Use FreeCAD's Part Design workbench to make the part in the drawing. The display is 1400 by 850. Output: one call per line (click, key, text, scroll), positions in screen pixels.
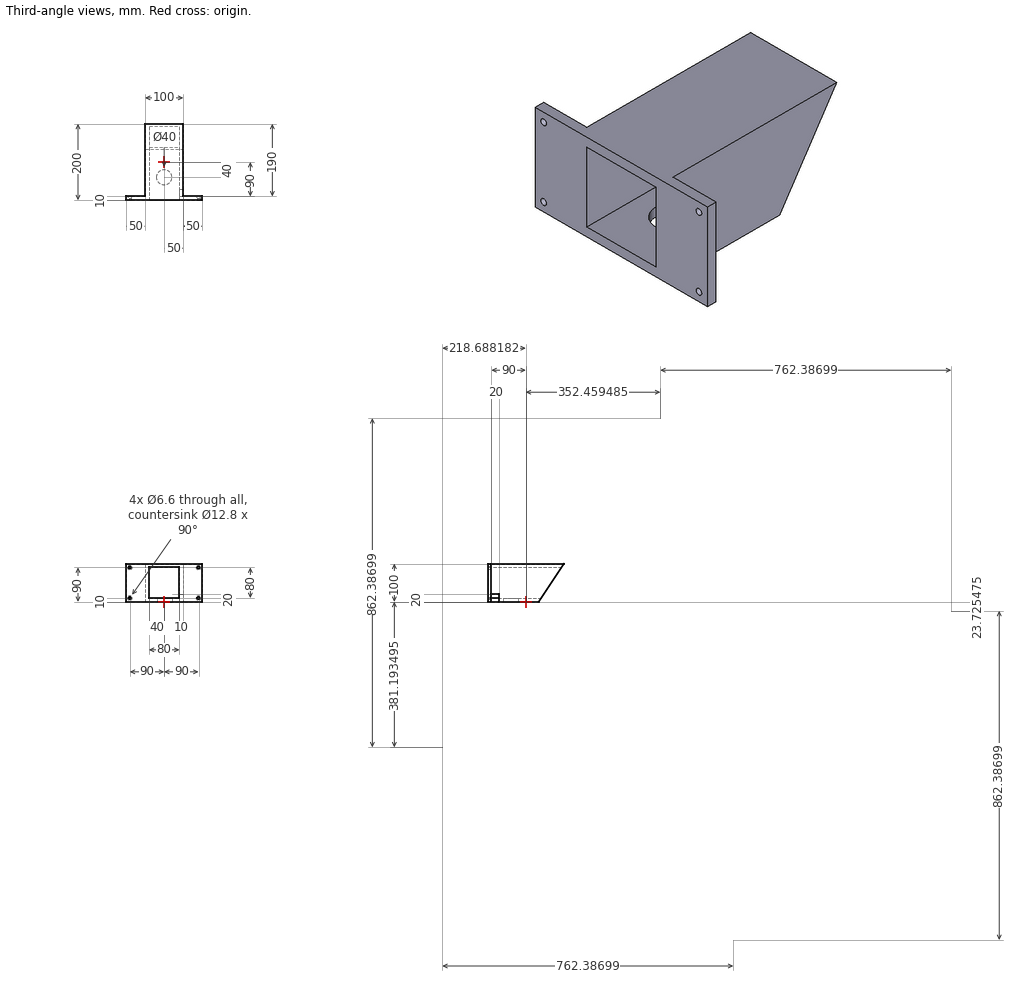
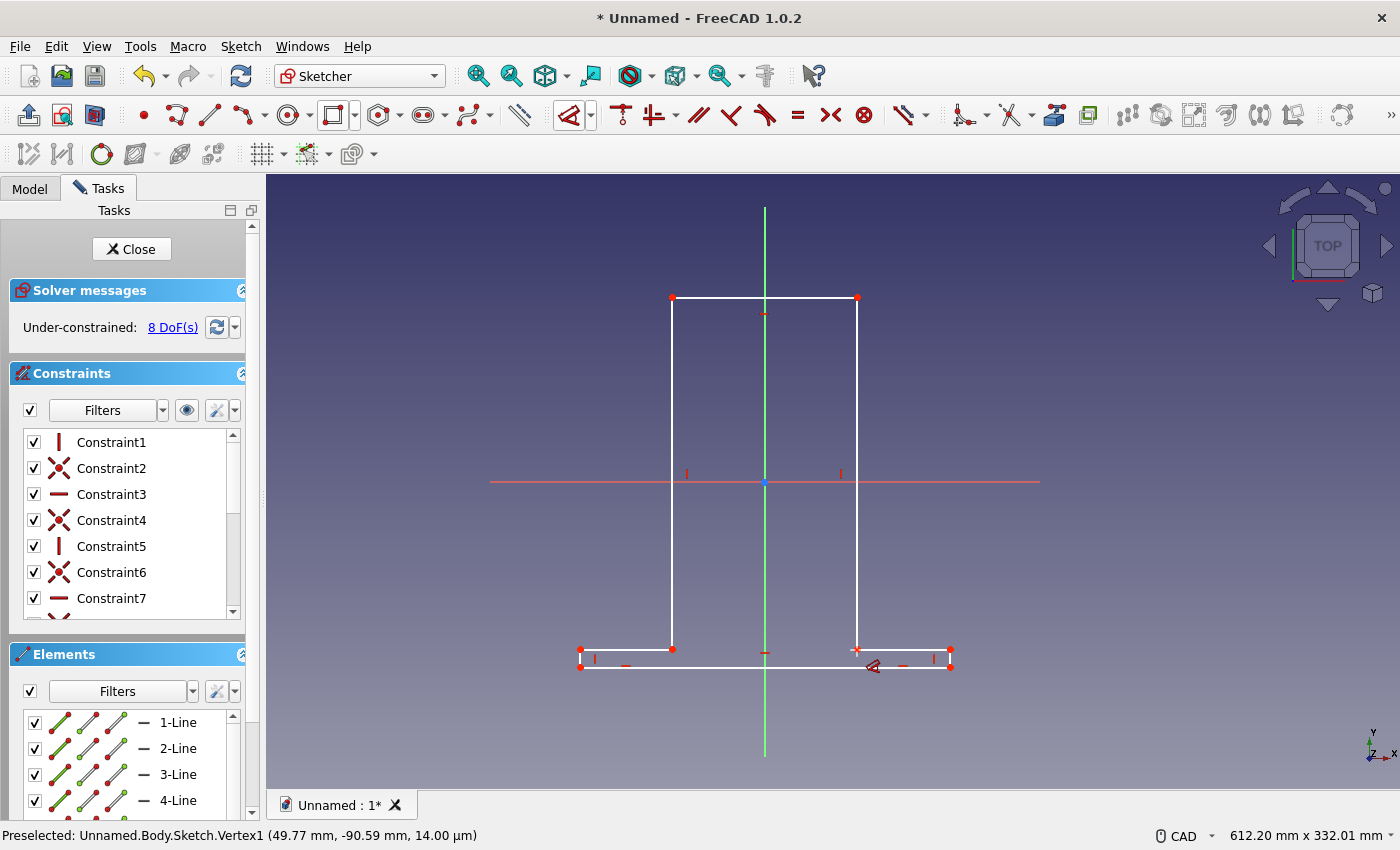
click(644, 650)
click(626, 684)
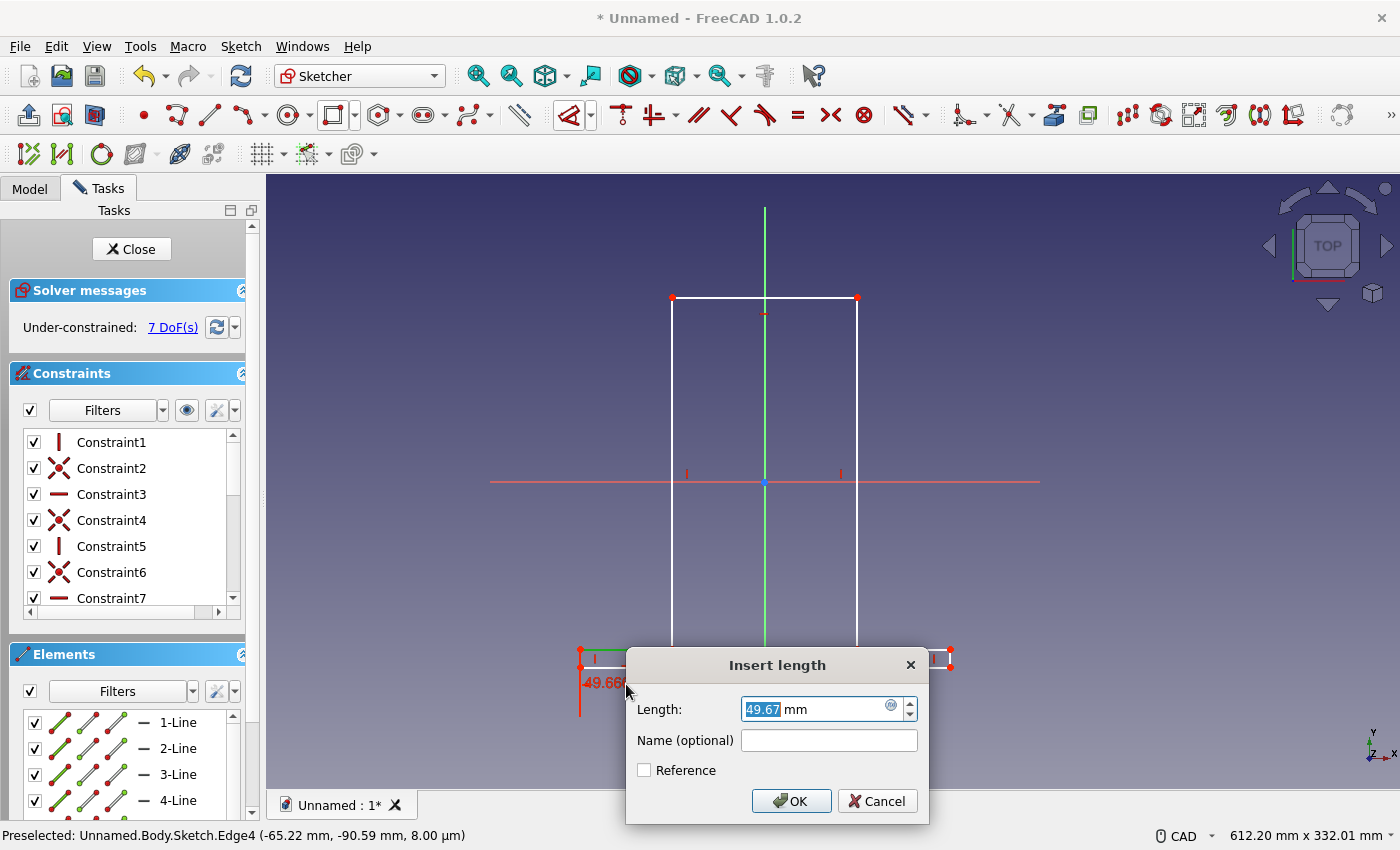
text(50)
key(Return)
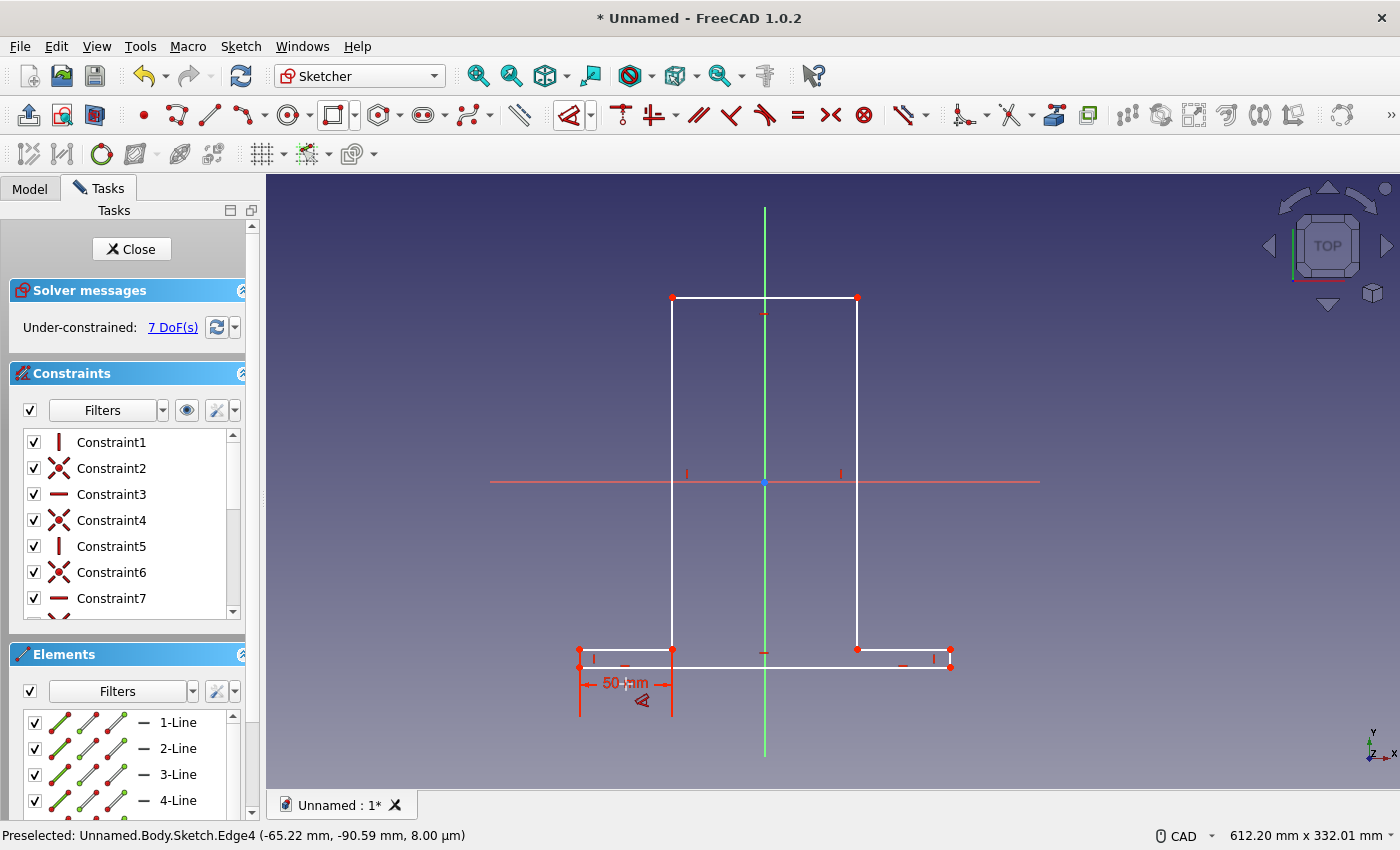
scroll(580, 659, up, 4)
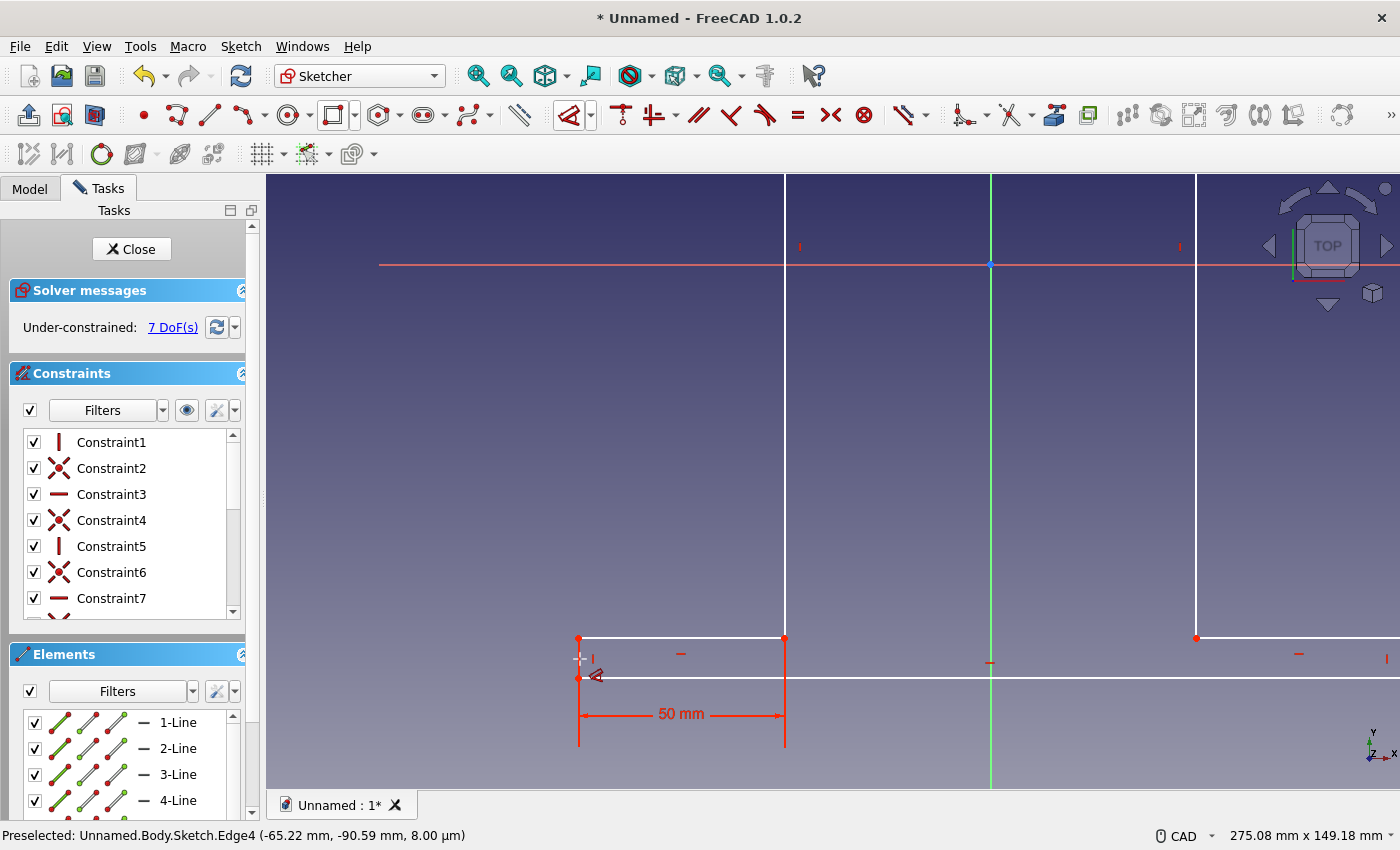
click(579, 658)
click(545, 658)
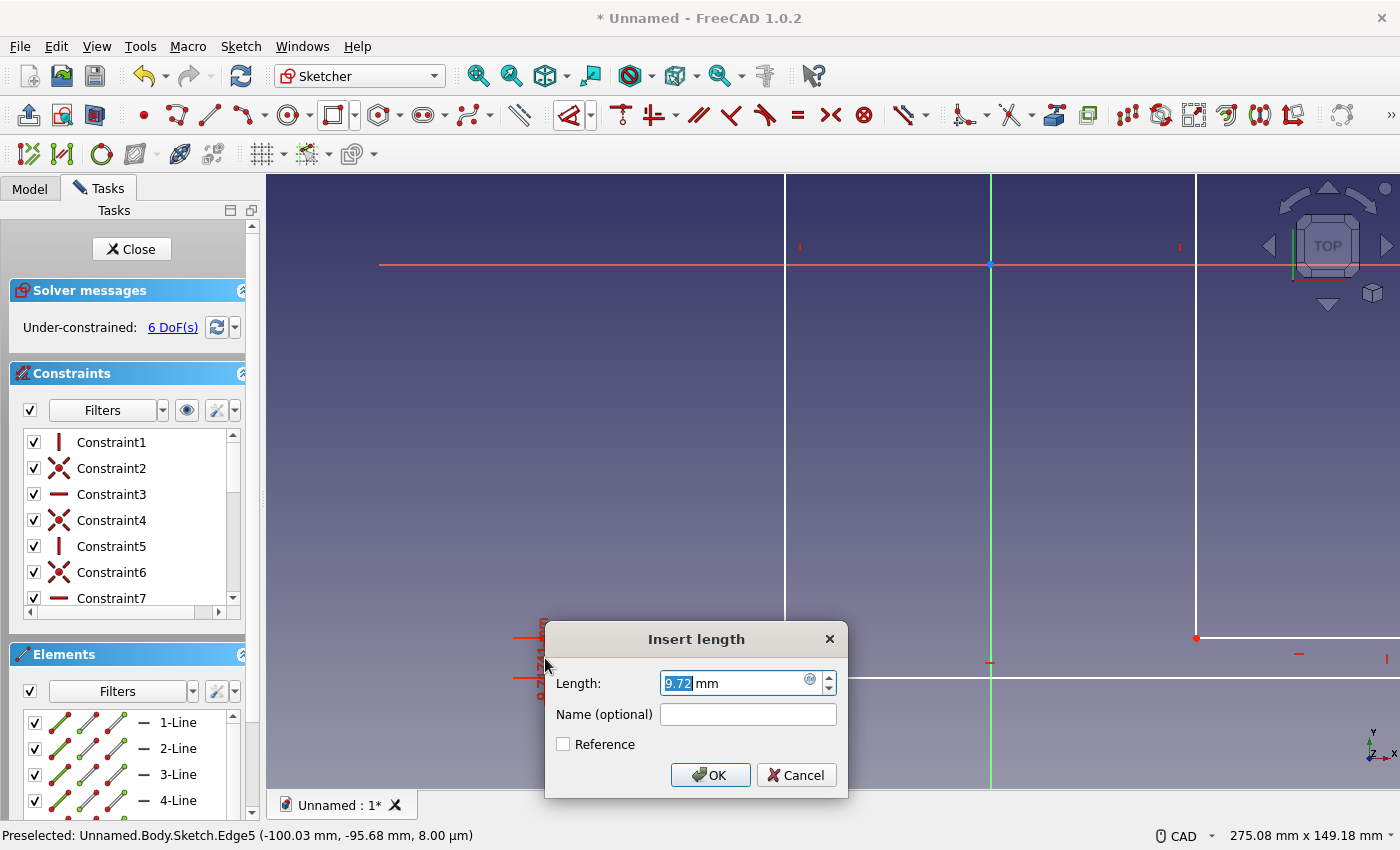
text(10)
key(Return)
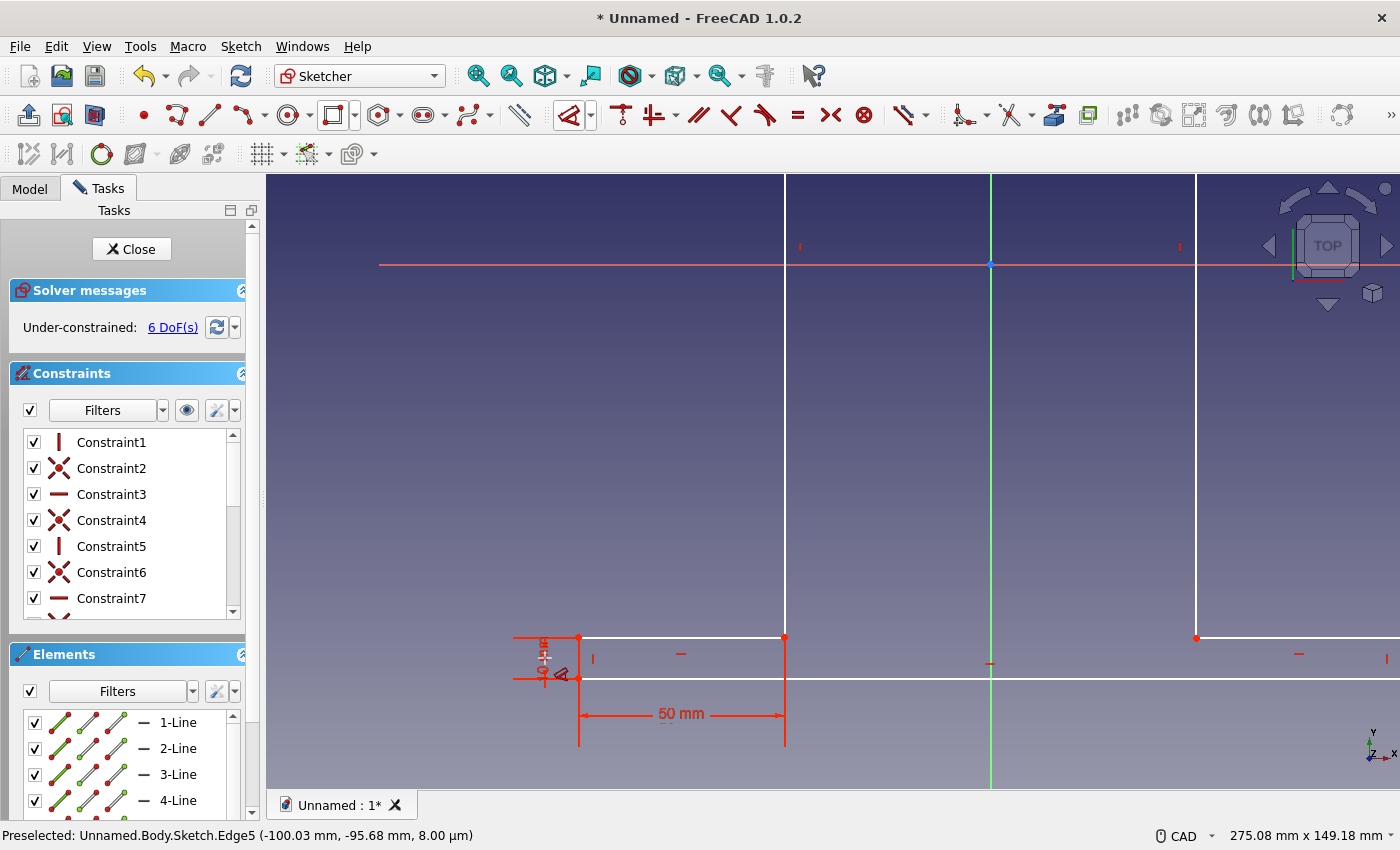
scroll(580, 659, down, 4)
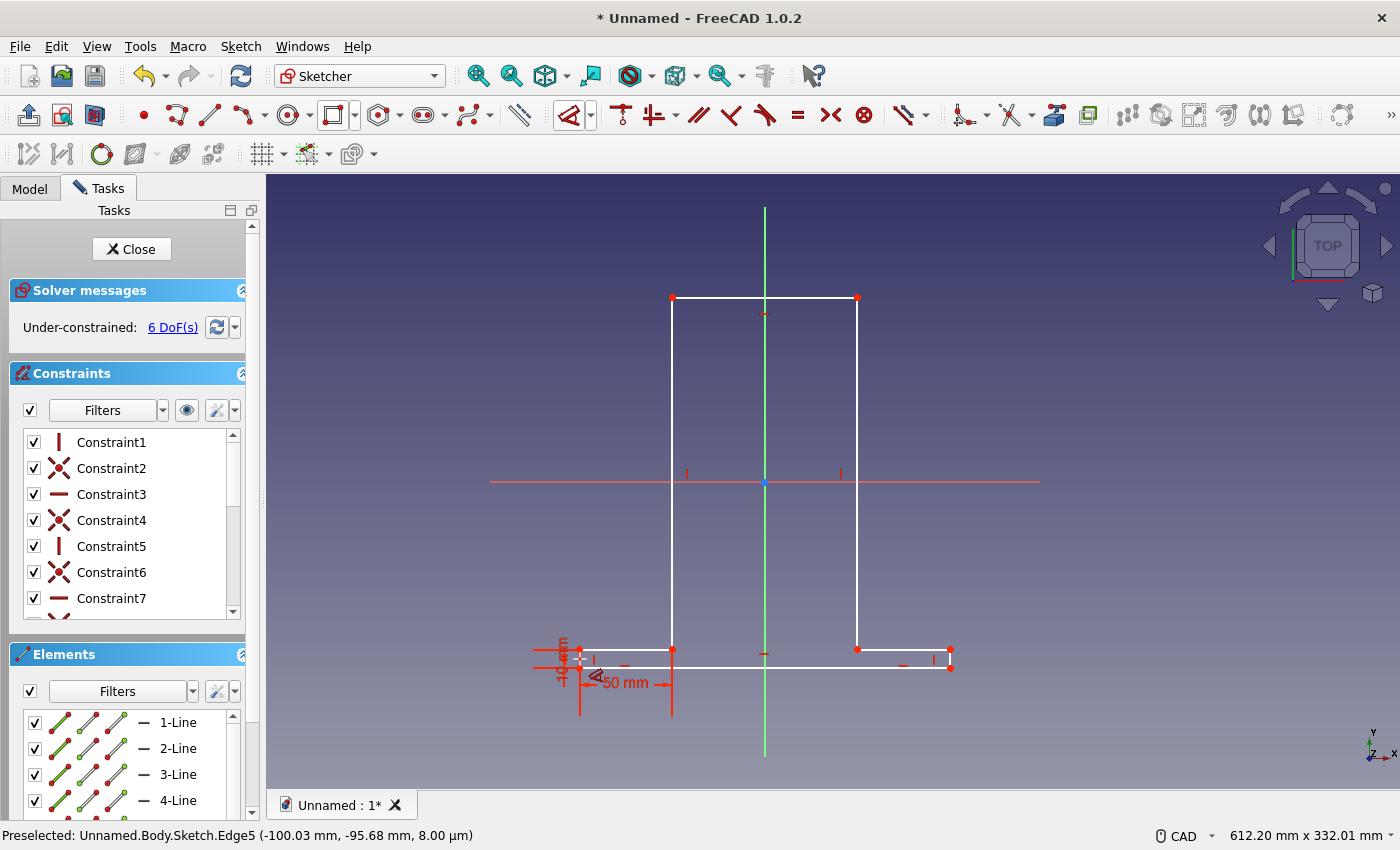
scroll(950, 663, up, 5)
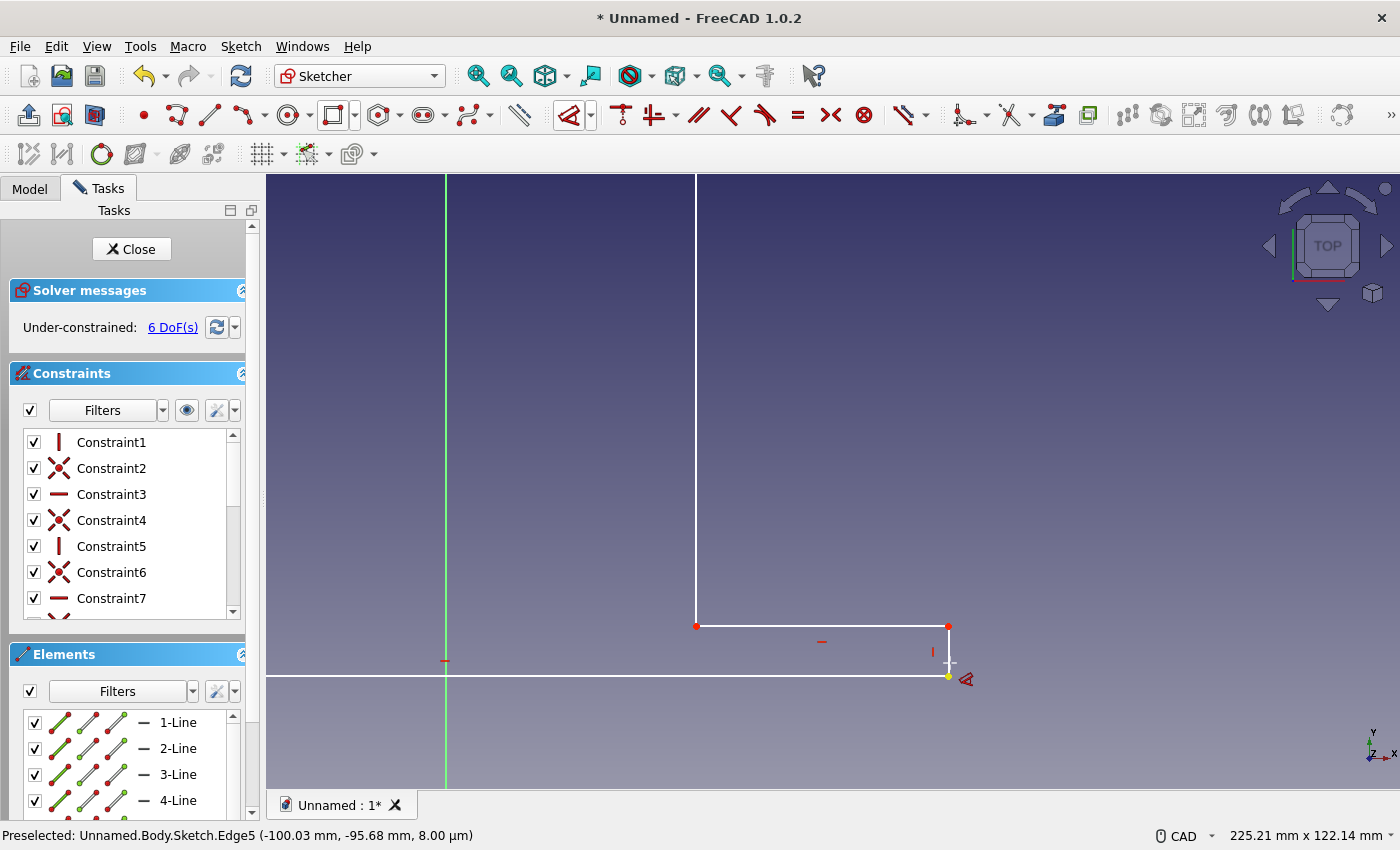
click(949, 661)
click(983, 651)